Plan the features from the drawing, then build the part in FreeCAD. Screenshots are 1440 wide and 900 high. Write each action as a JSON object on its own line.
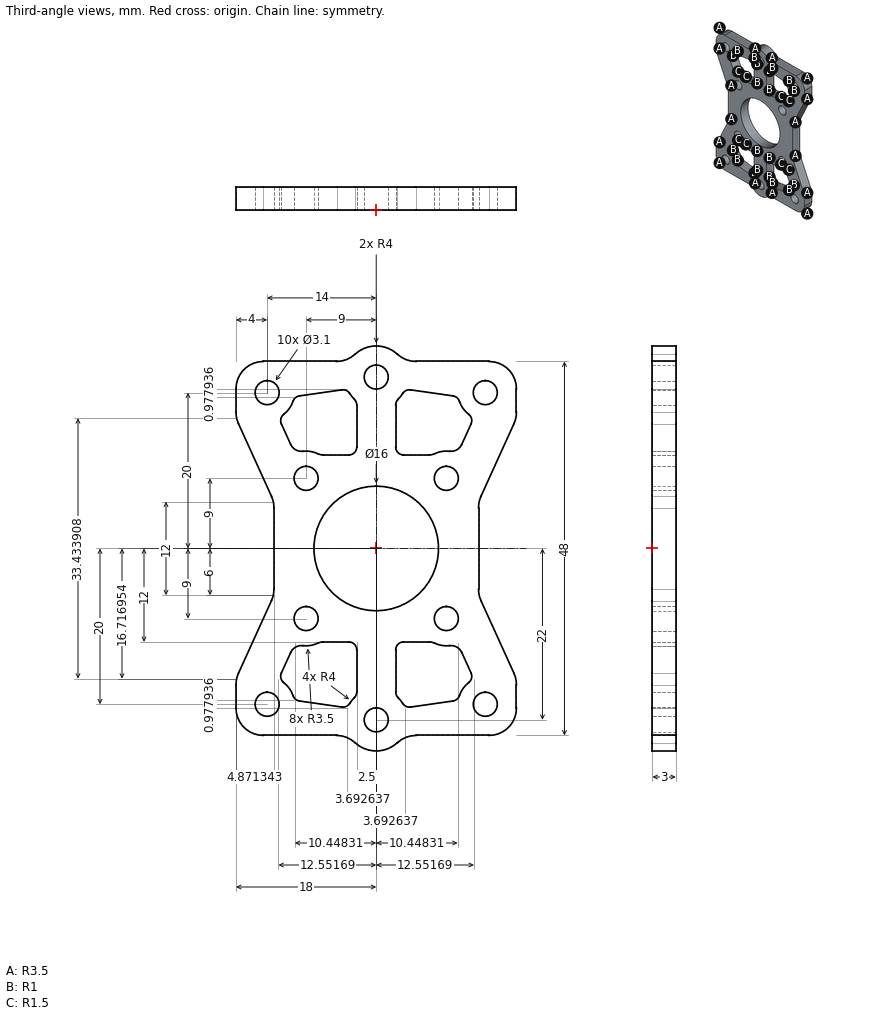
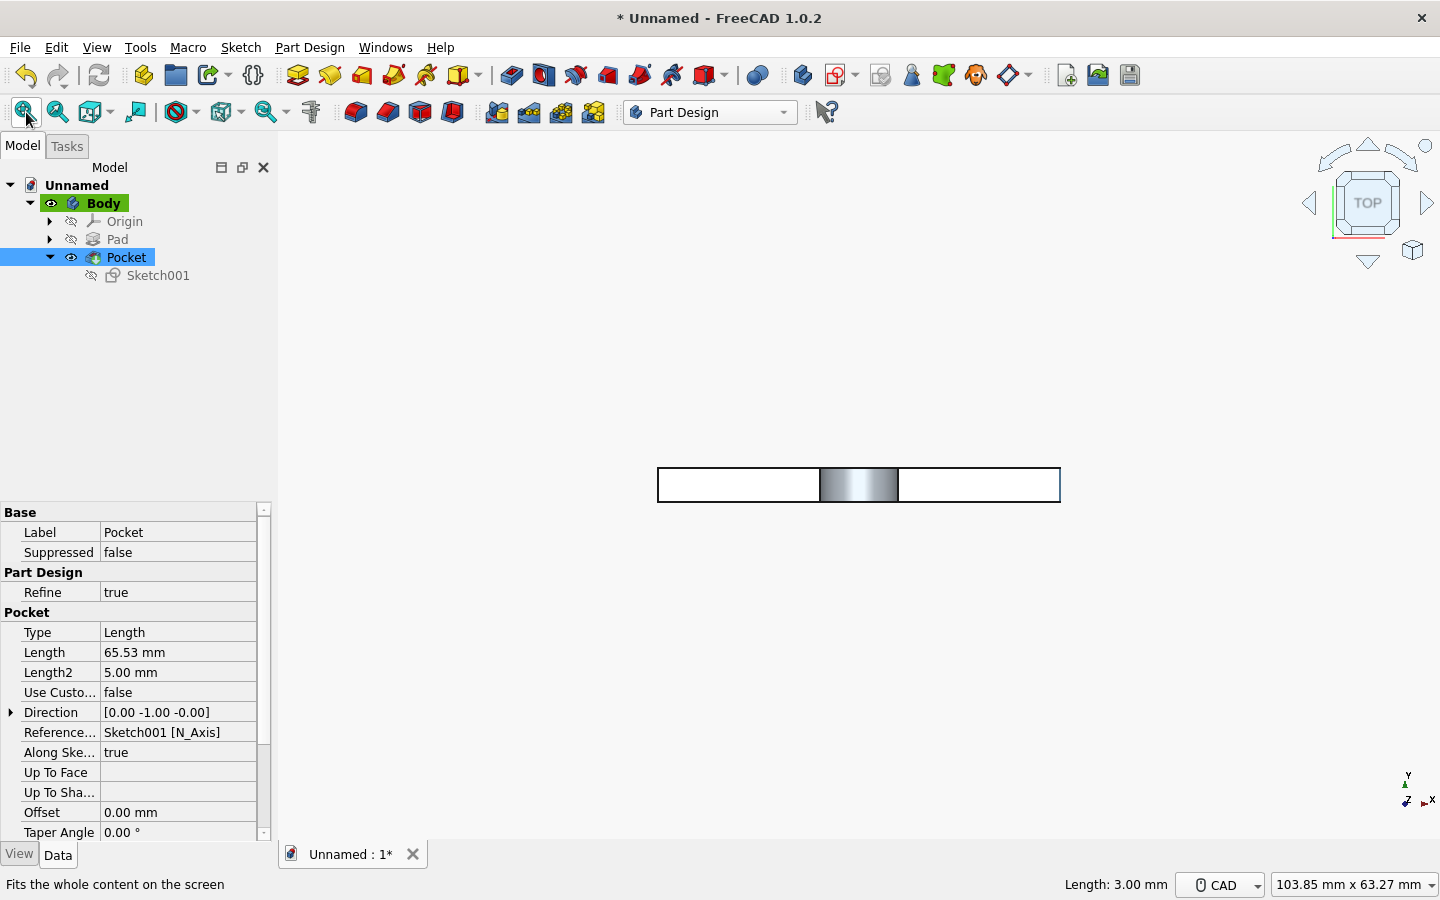
{"action": "left_click", "coordinate": [658, 484], "text": "ctrl"}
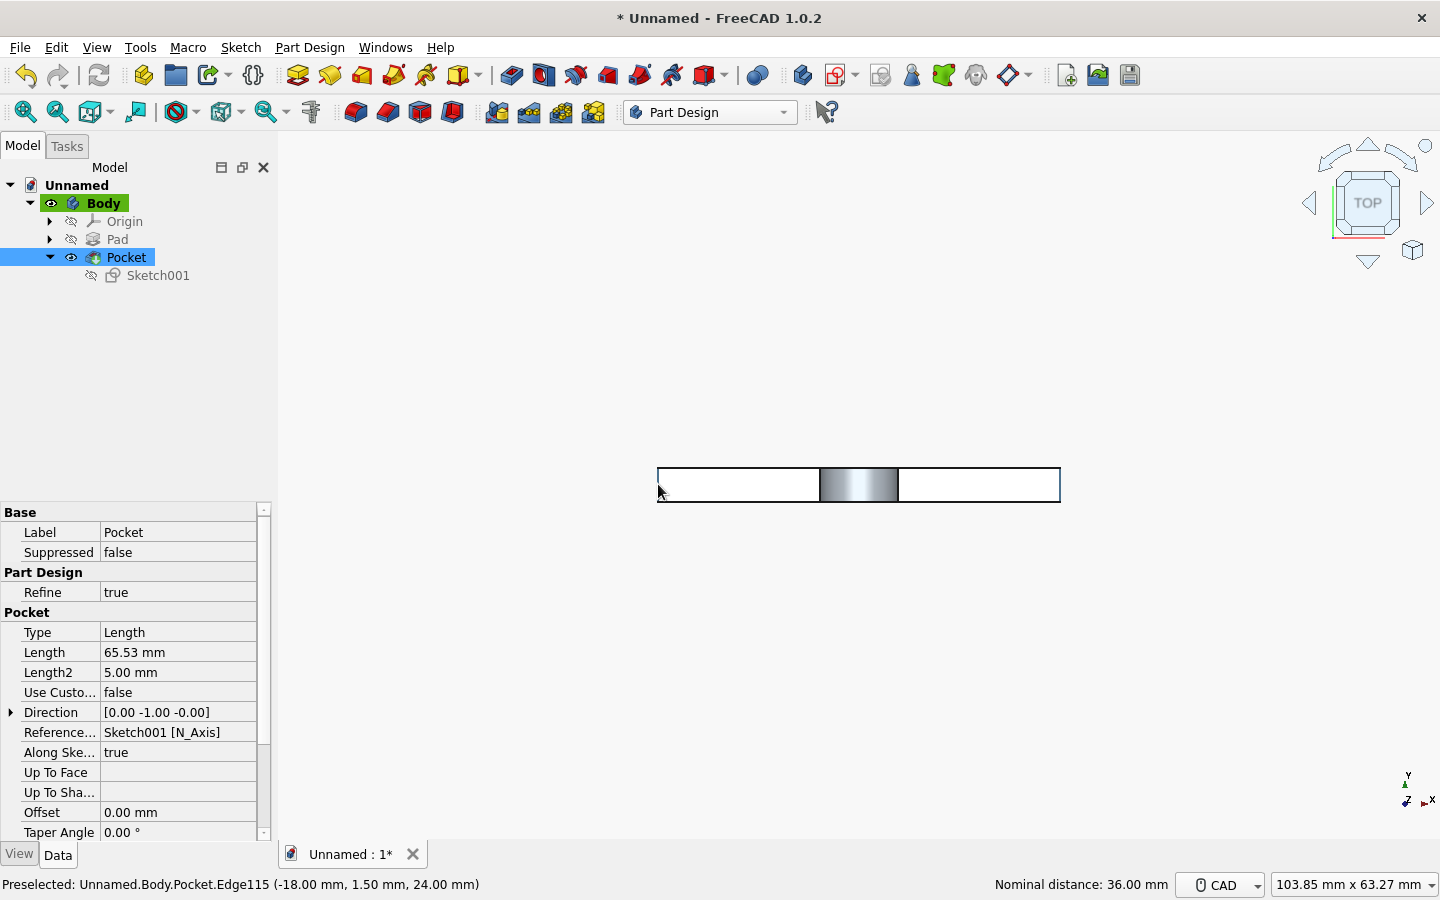
{"action": "key", "text": "1"}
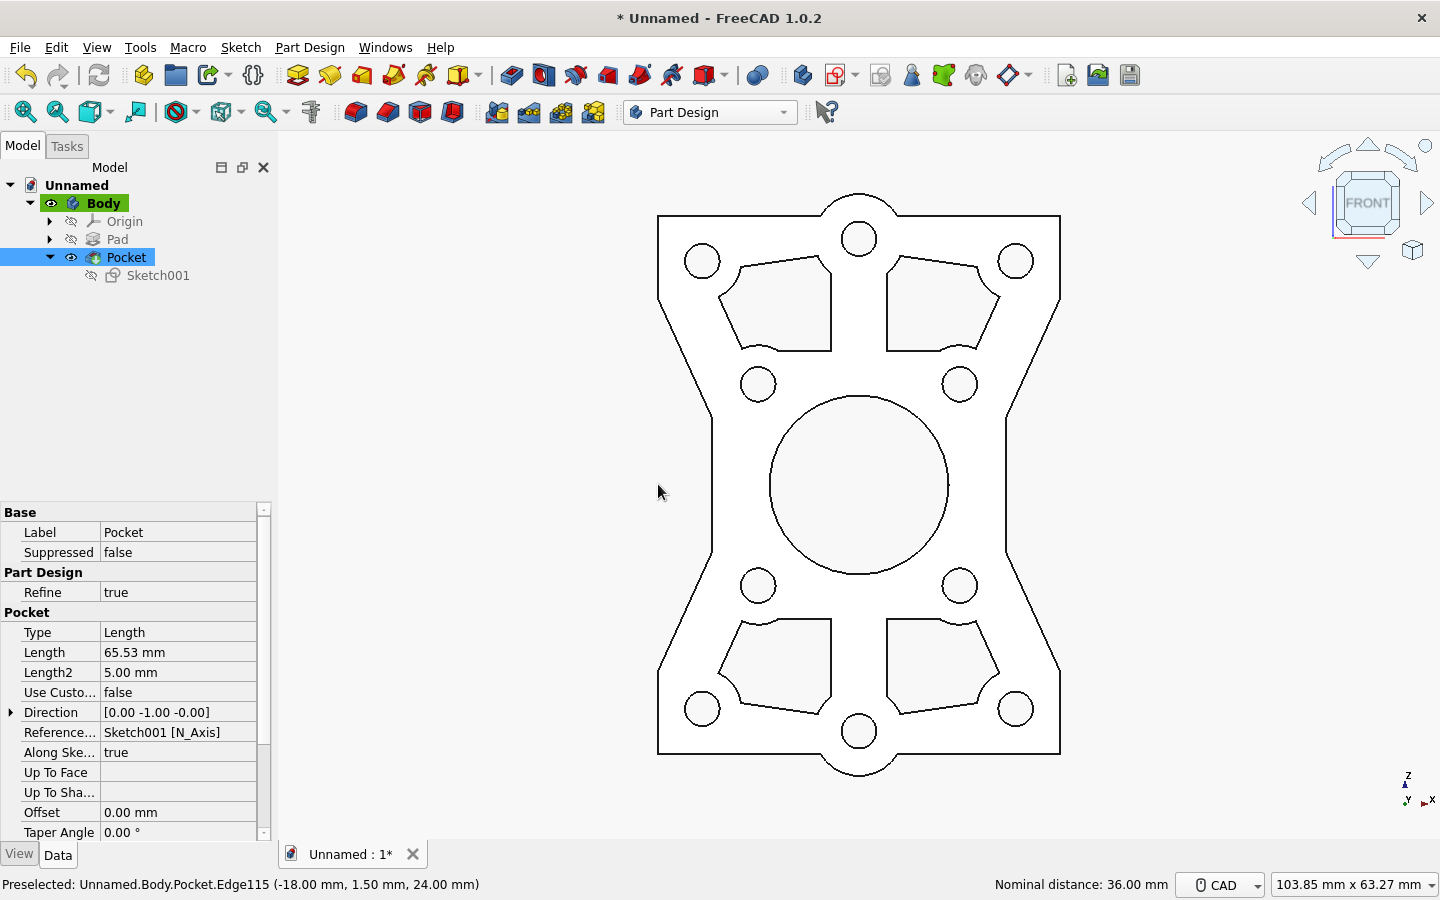
{"action": "key", "text": "3"}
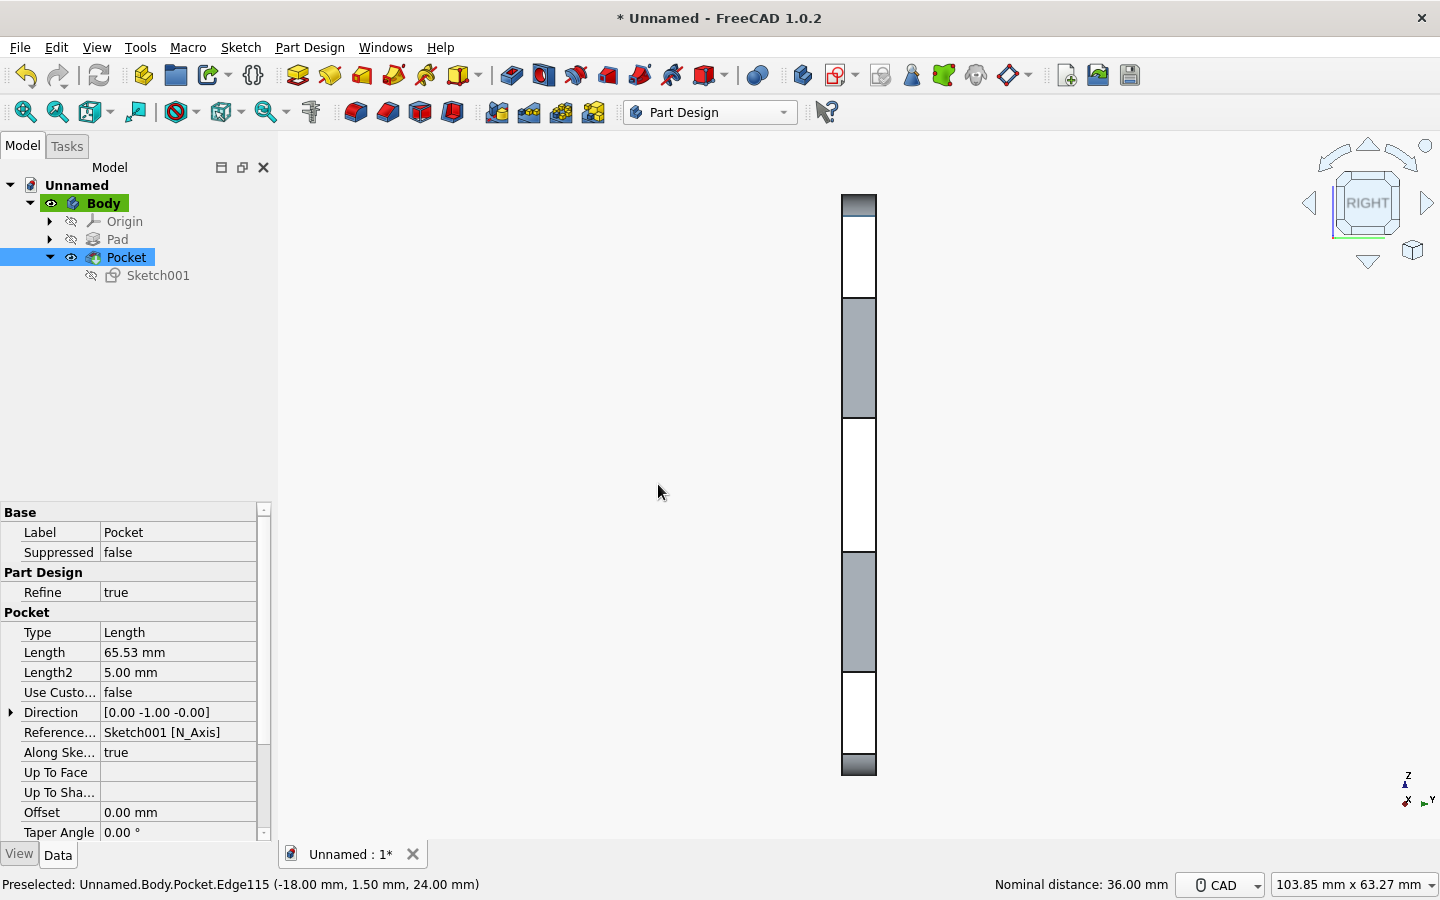
{"action": "left_click", "coordinate": [859, 671], "text": "ctrl"}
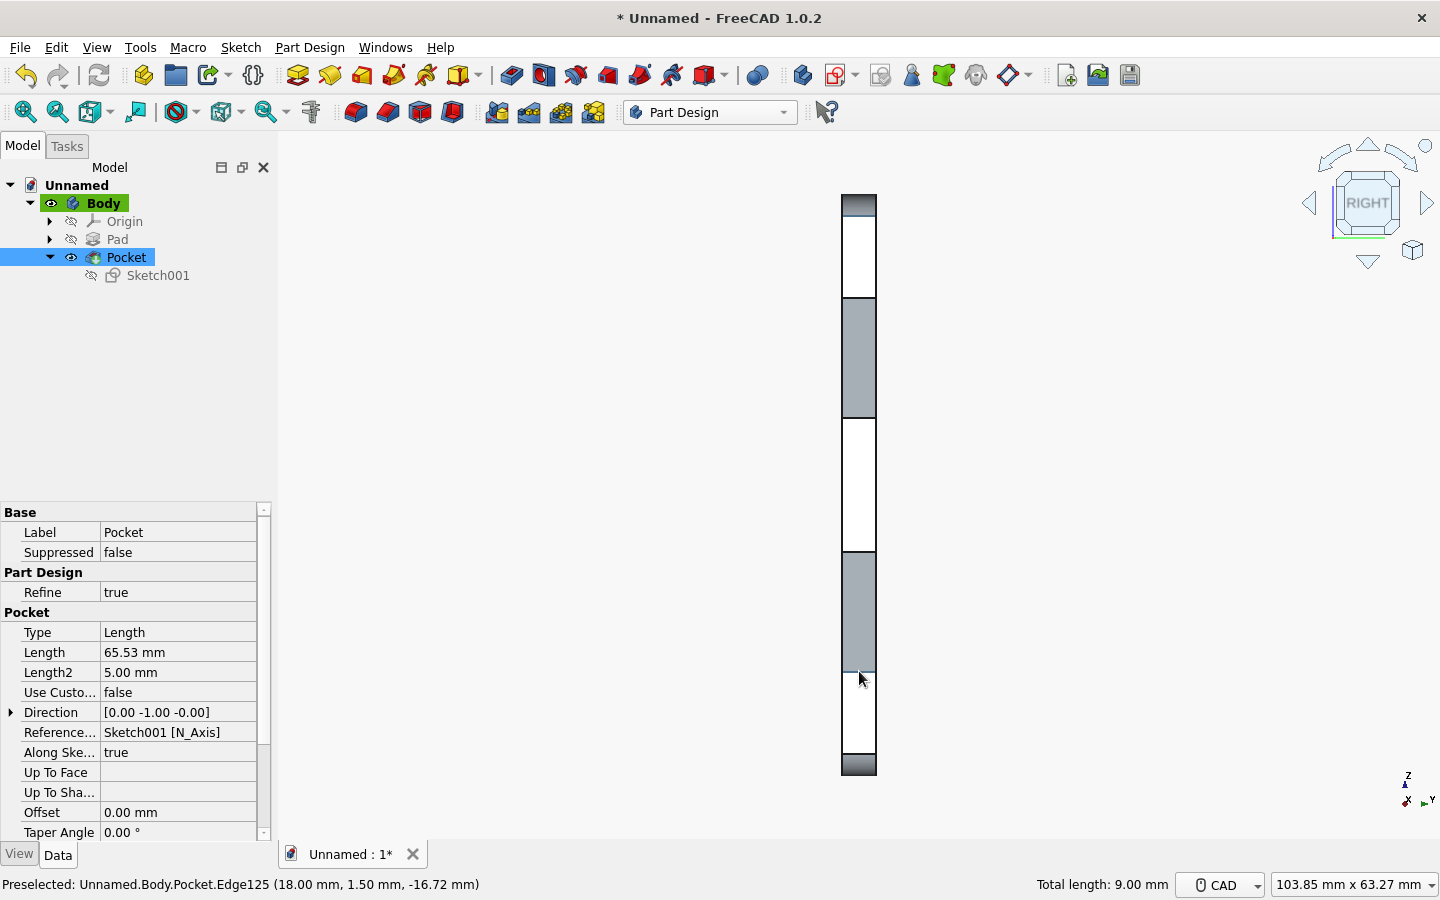
{"action": "left_click", "coordinate": [859, 297], "text": "ctrl"}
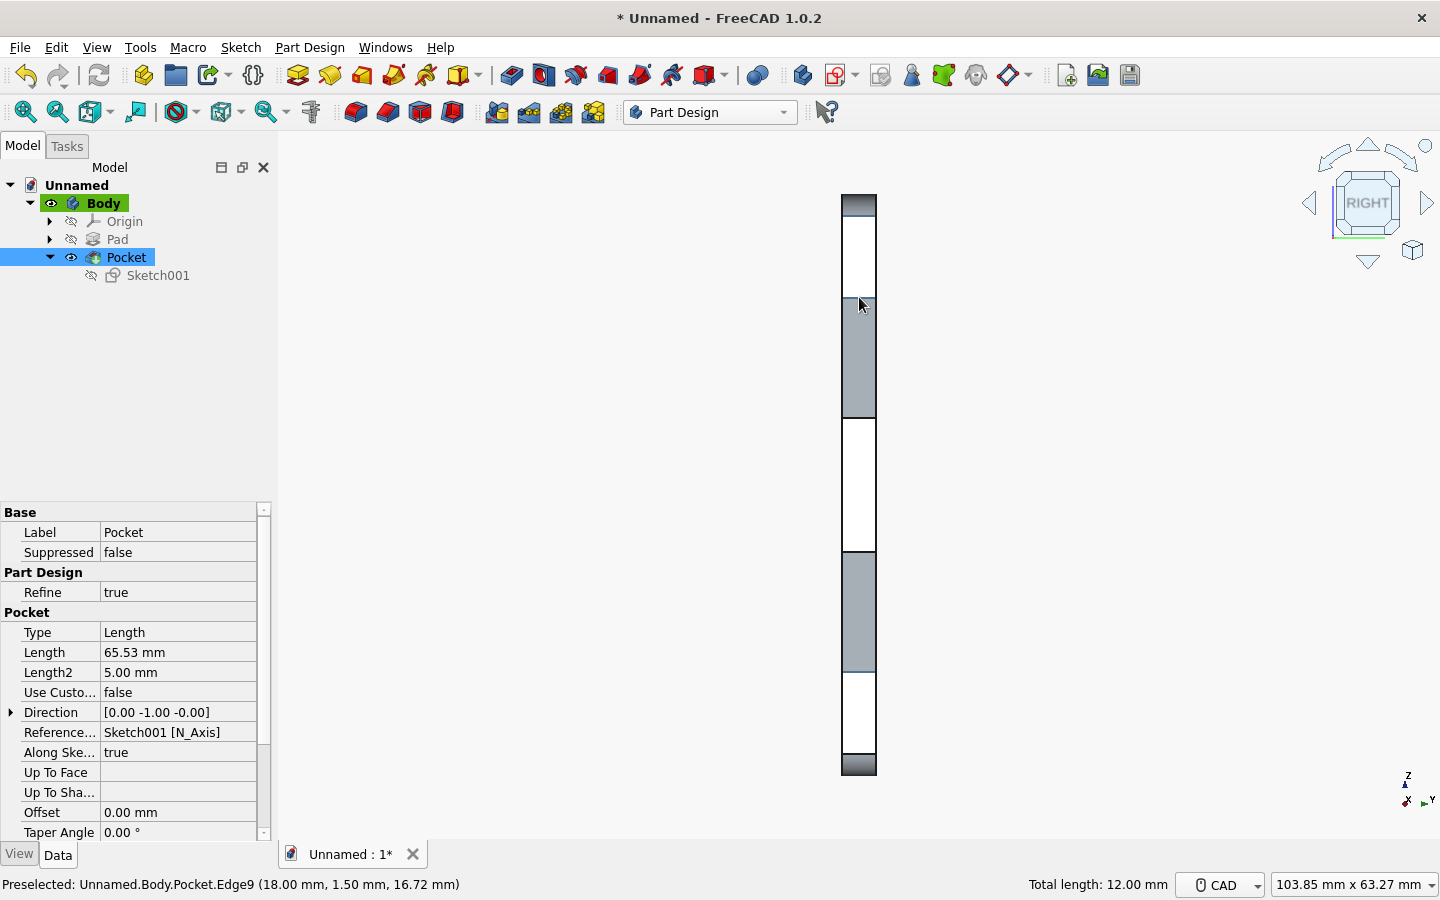
{"action": "left_click", "coordinate": [859, 753], "text": "ctrl"}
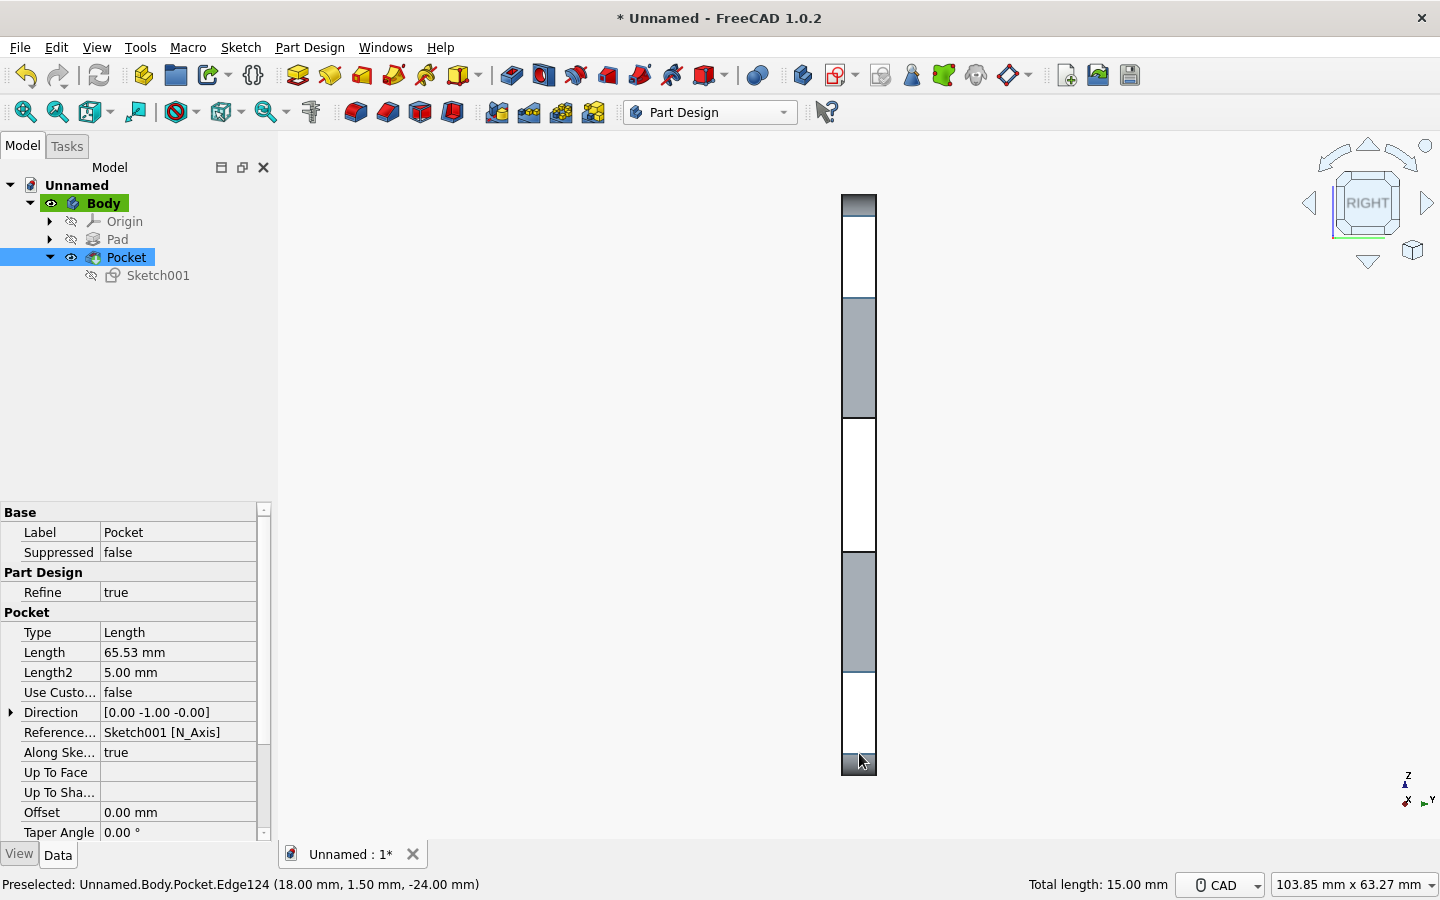
{"action": "key", "text": "5"}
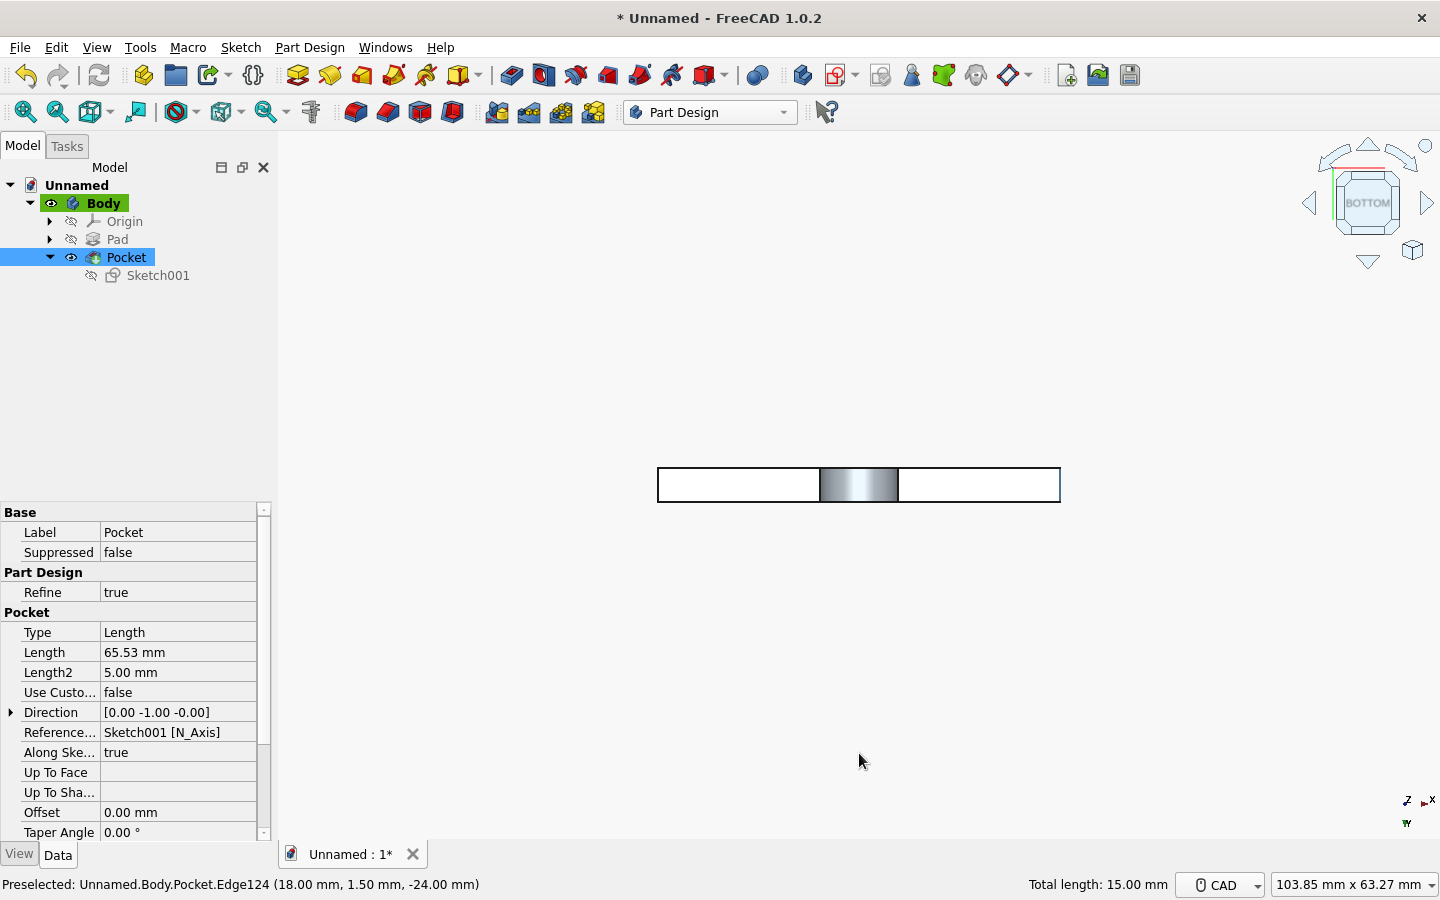
{"action": "left_click", "coordinate": [26, 112]}